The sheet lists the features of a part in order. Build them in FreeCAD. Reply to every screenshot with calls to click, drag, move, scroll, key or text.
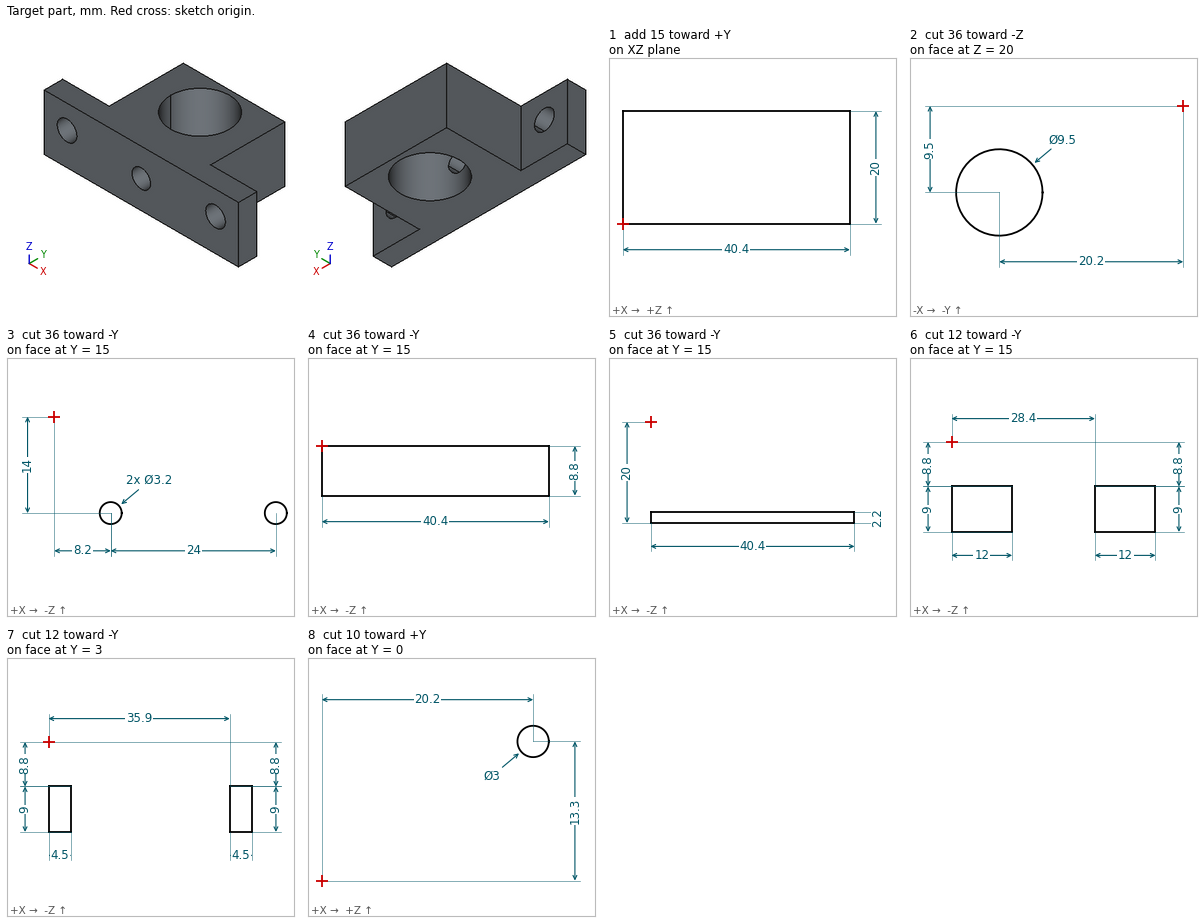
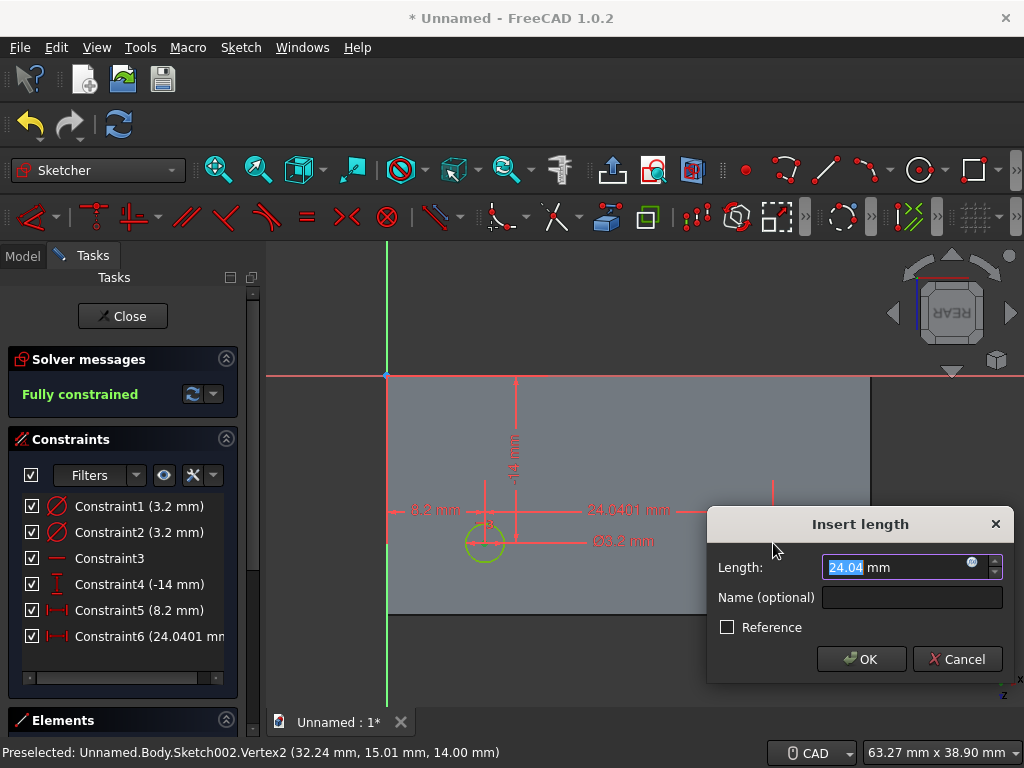
text(24)
key(Return)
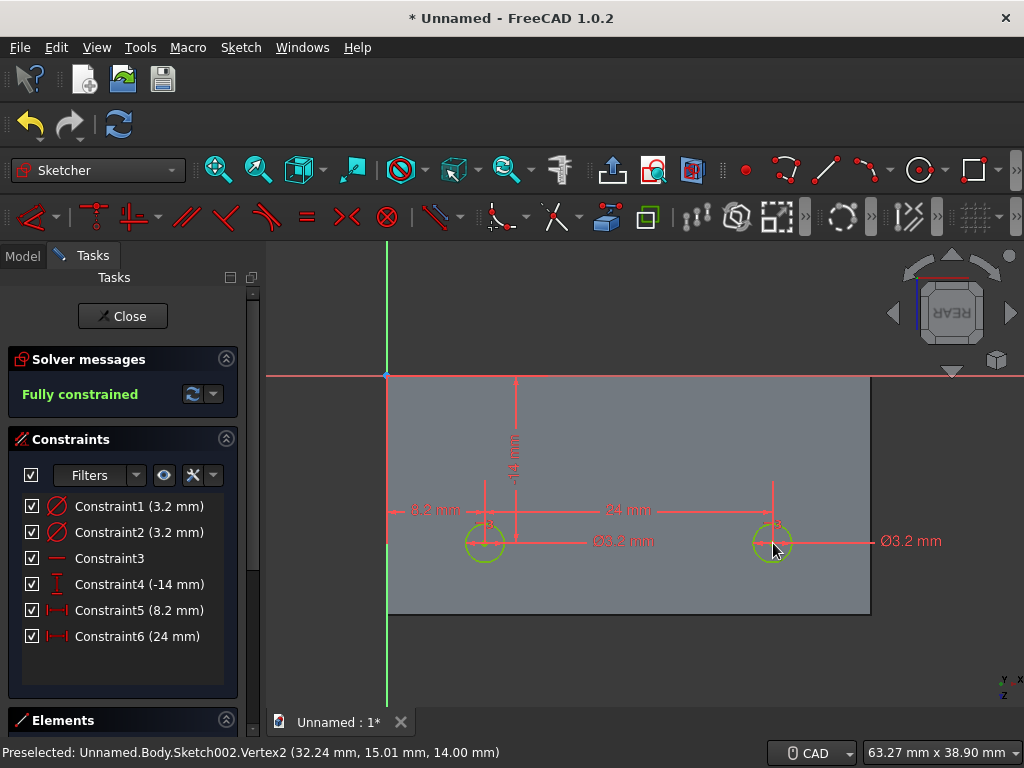
click(123, 316)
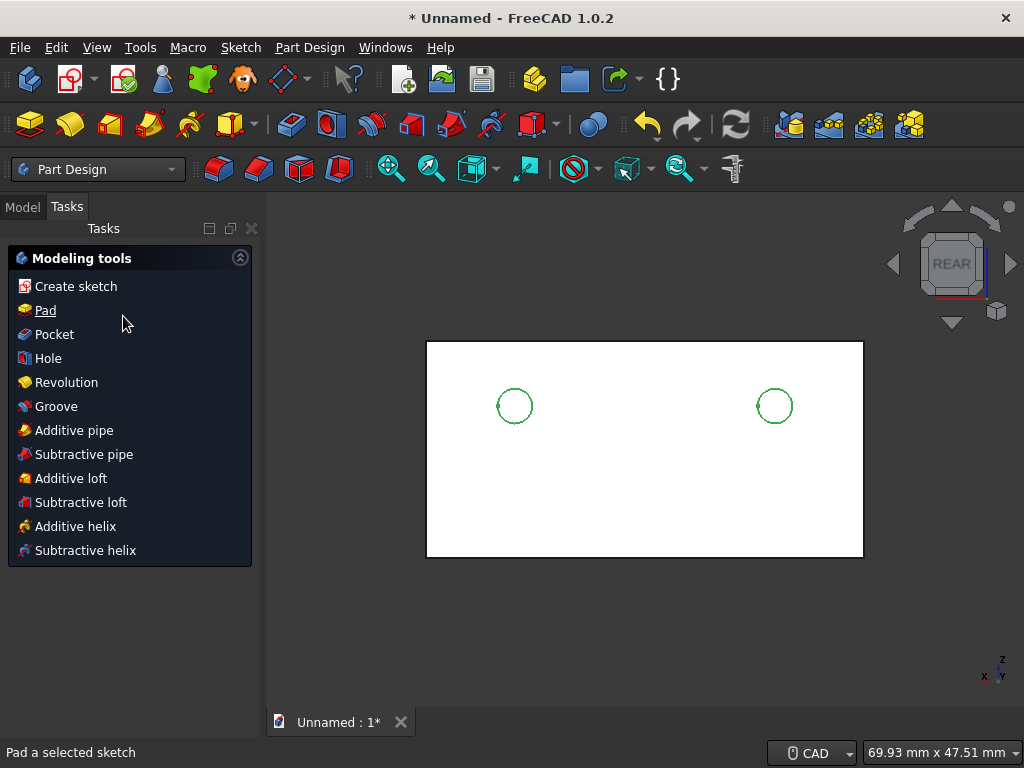
click(292, 124)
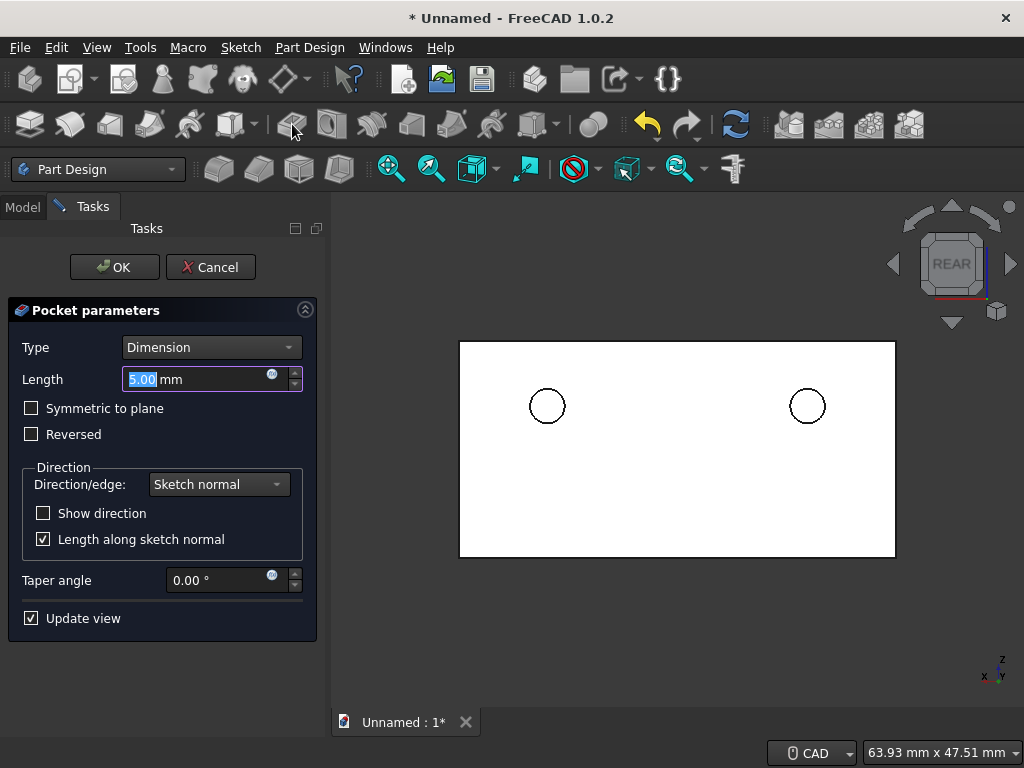
text(36)
key(Tab)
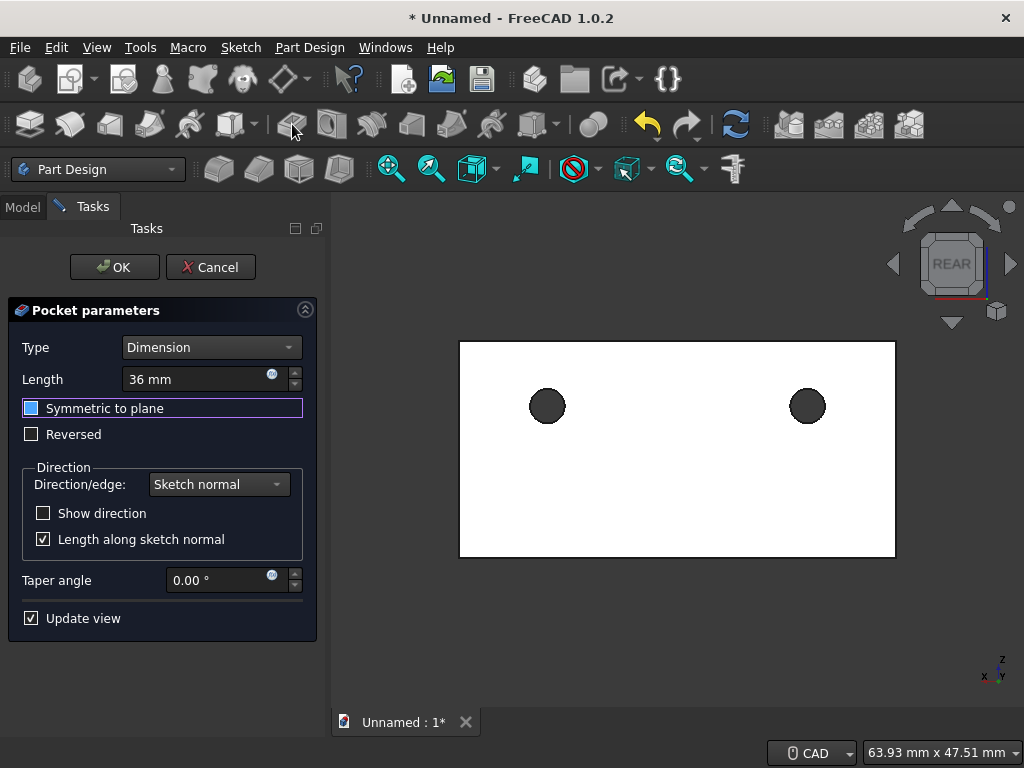
click(115, 267)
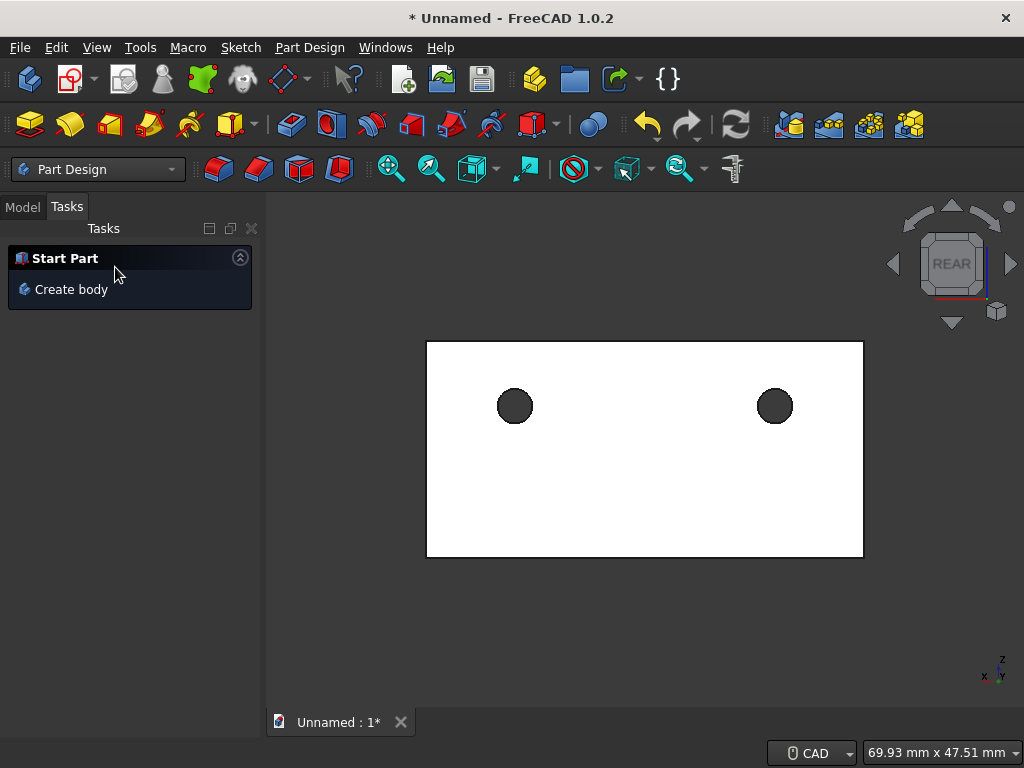
click(645, 449)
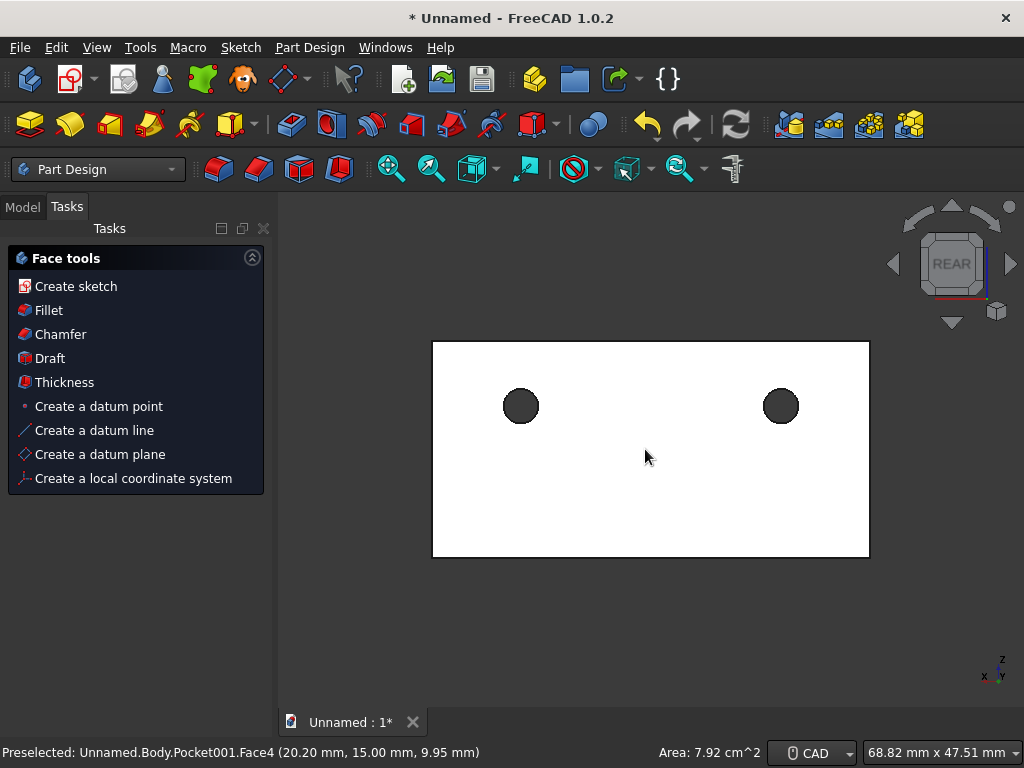
click(70, 80)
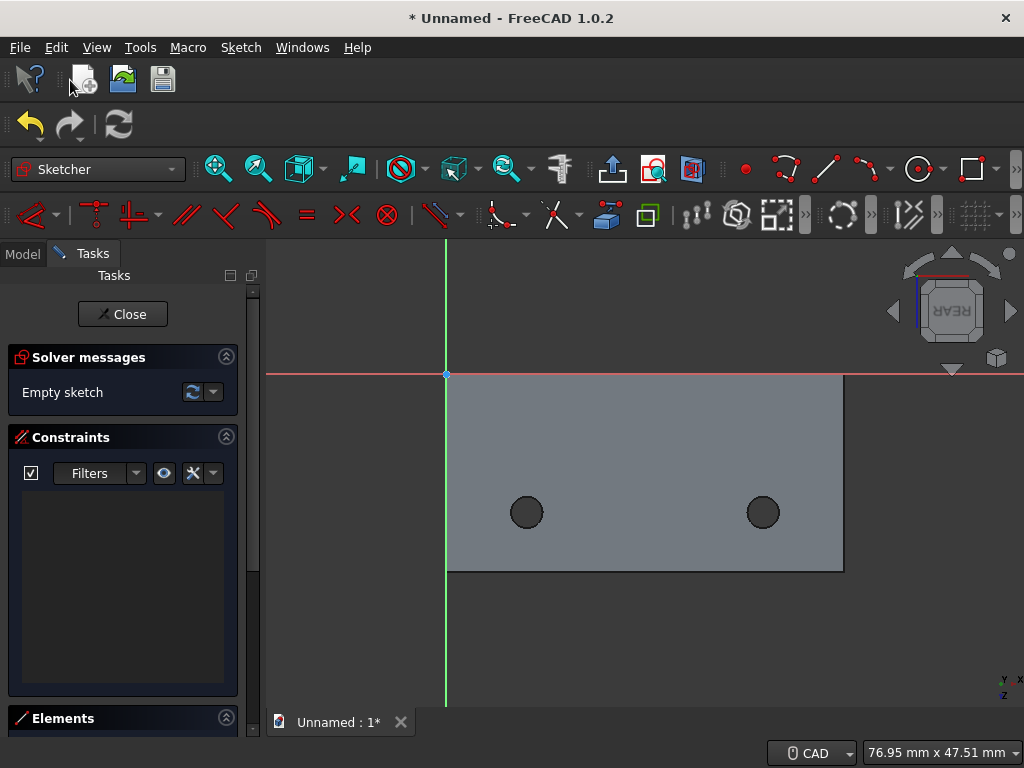
scroll(294, 679, down, 1)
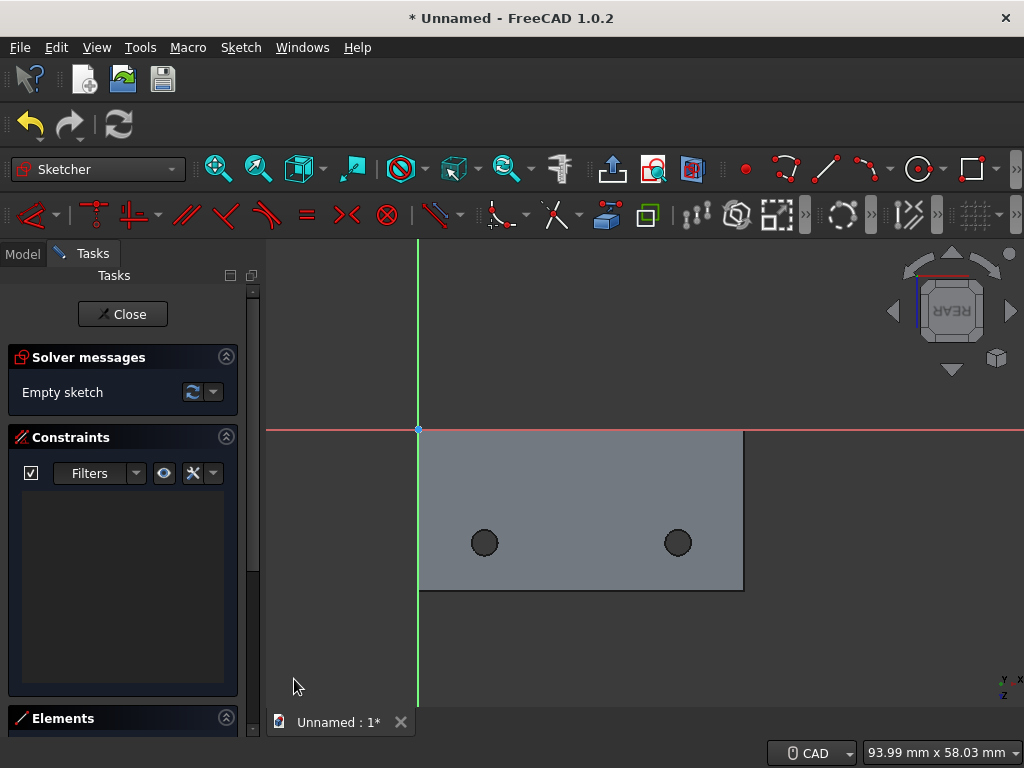
key(g)
key(r)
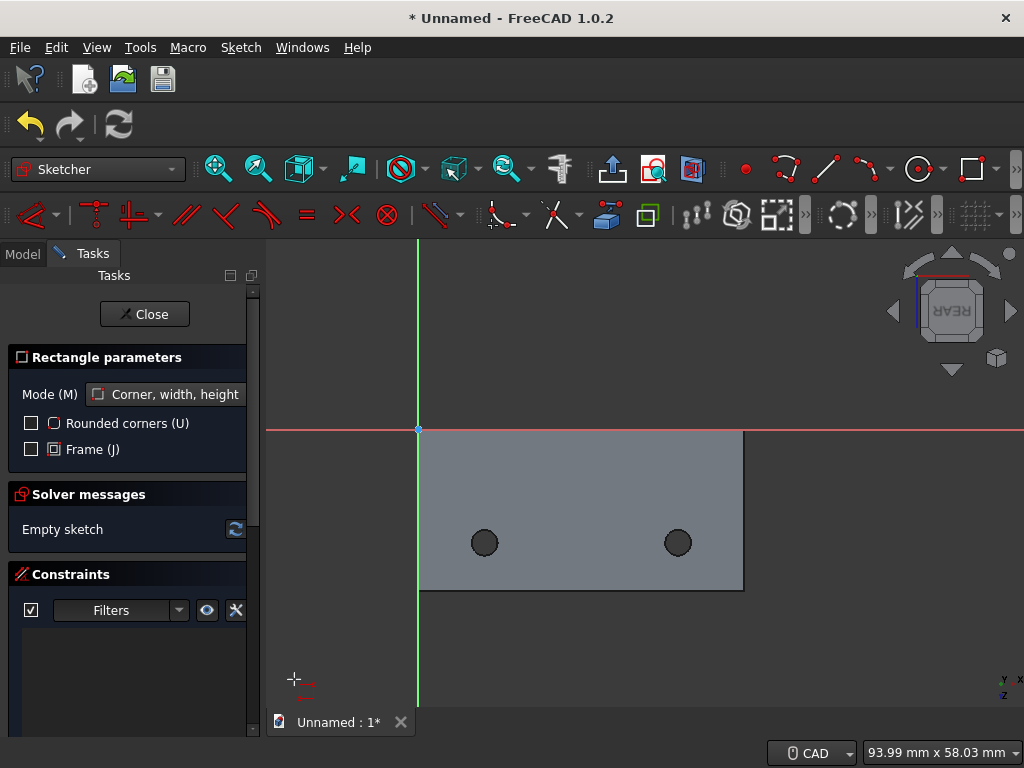
click(418, 430)
move(744, 501)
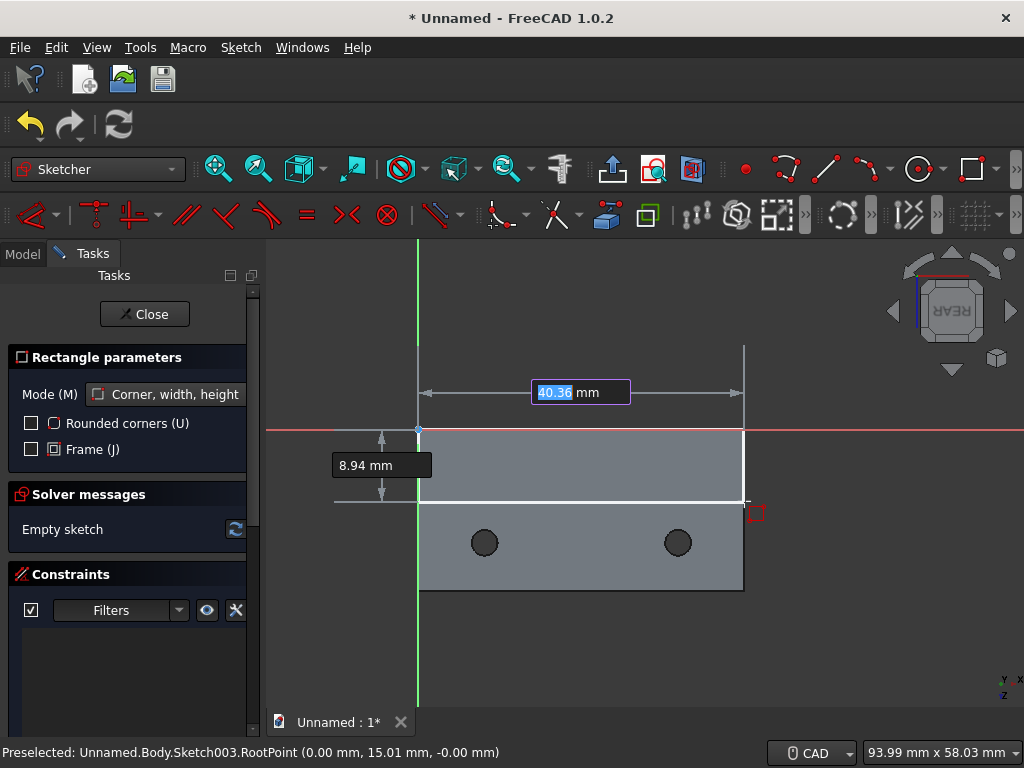
text(40.4)
key(Tab)
text(8.8)
key(Return)
key(Escape)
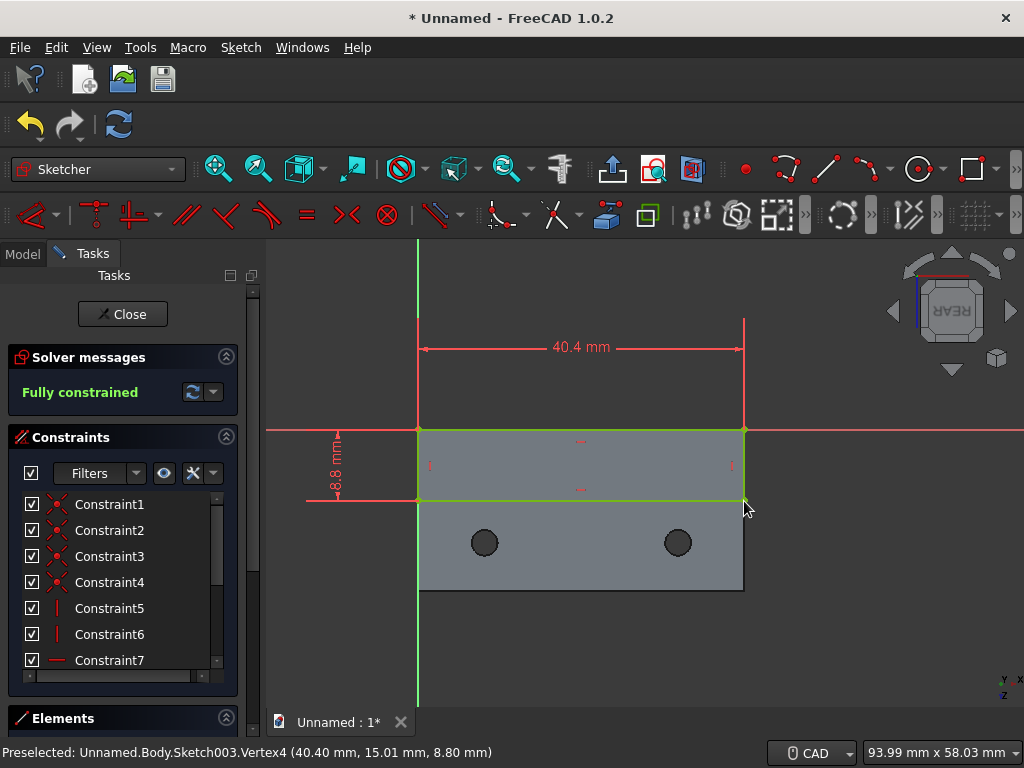
click(123, 314)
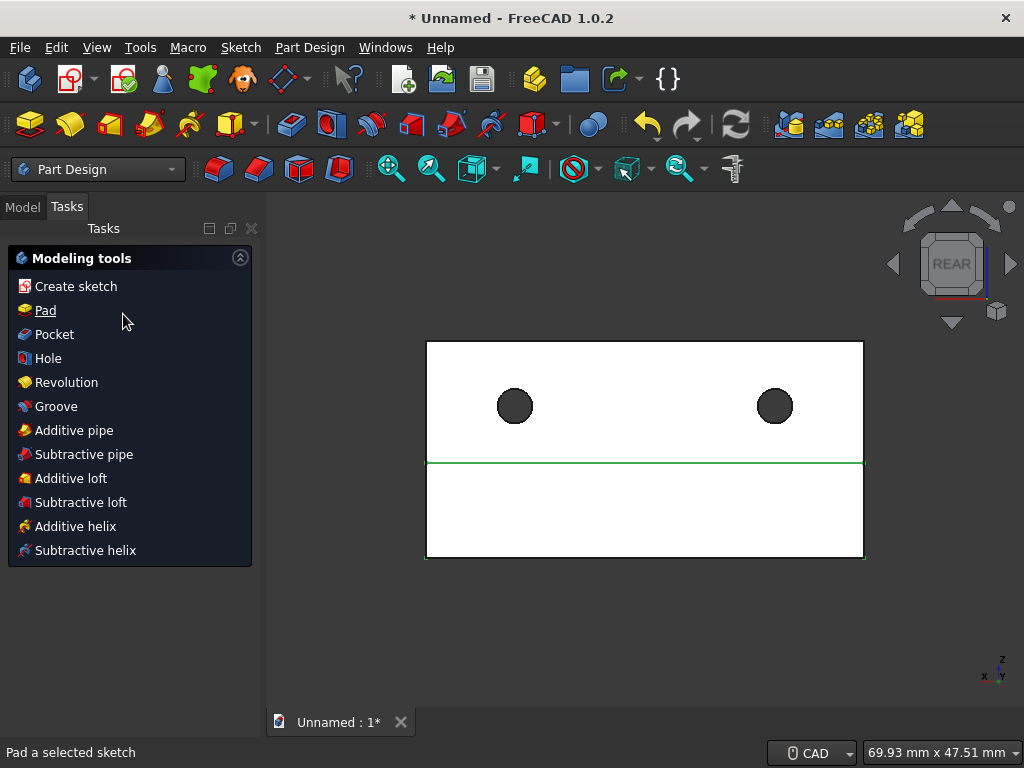
click(292, 124)